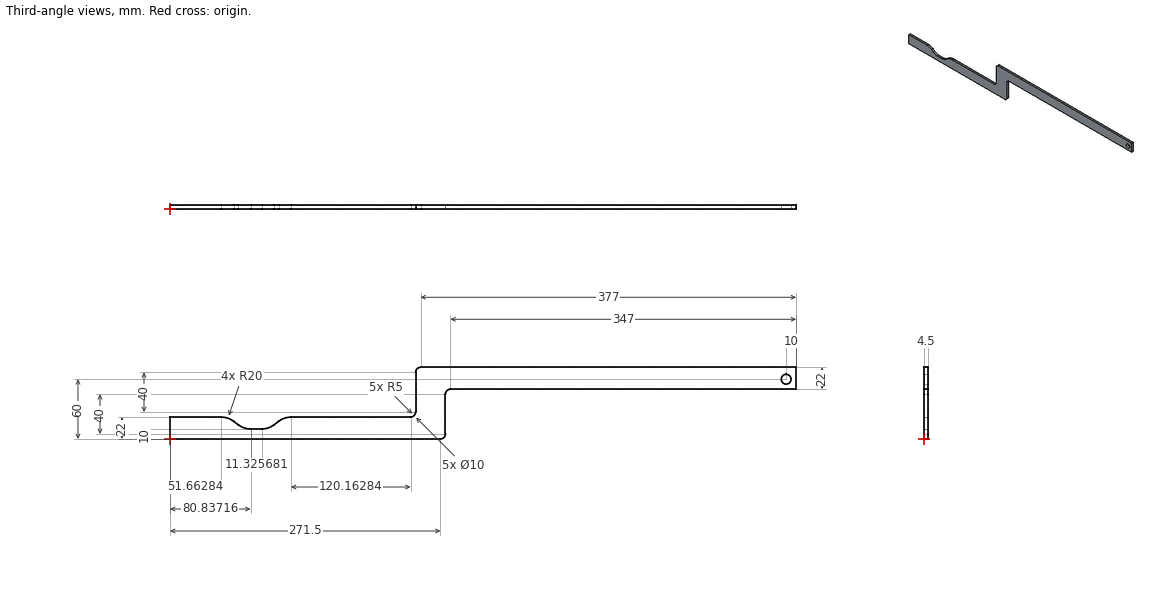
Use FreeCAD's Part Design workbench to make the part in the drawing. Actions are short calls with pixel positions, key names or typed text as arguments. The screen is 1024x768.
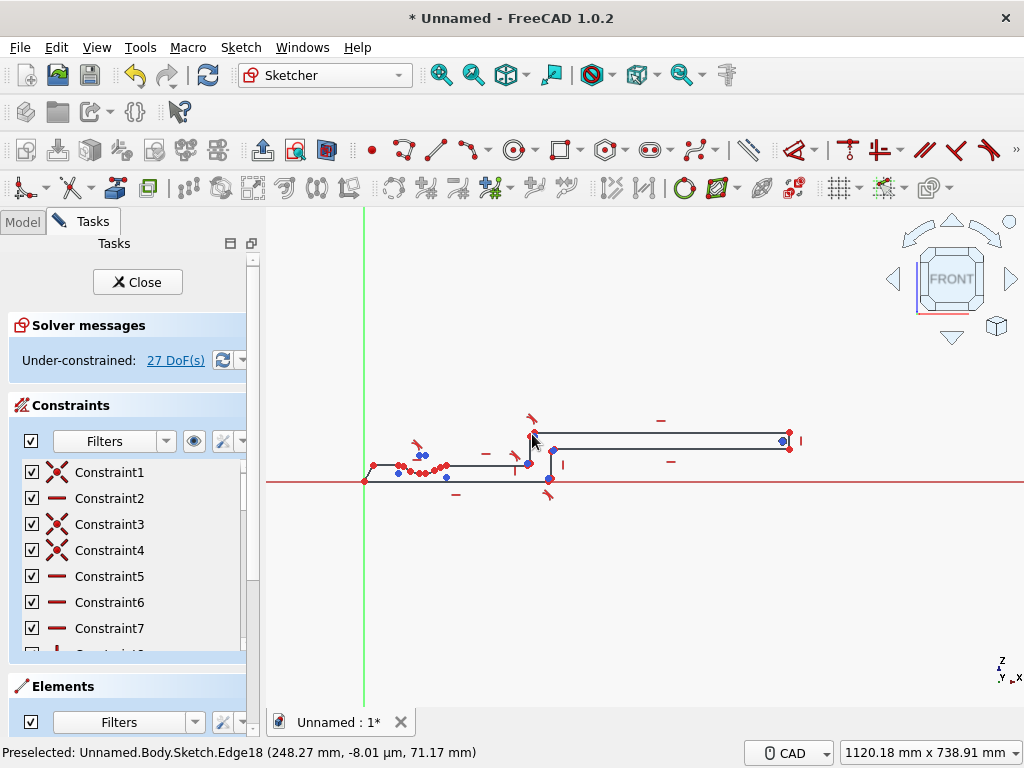
click(719, 449)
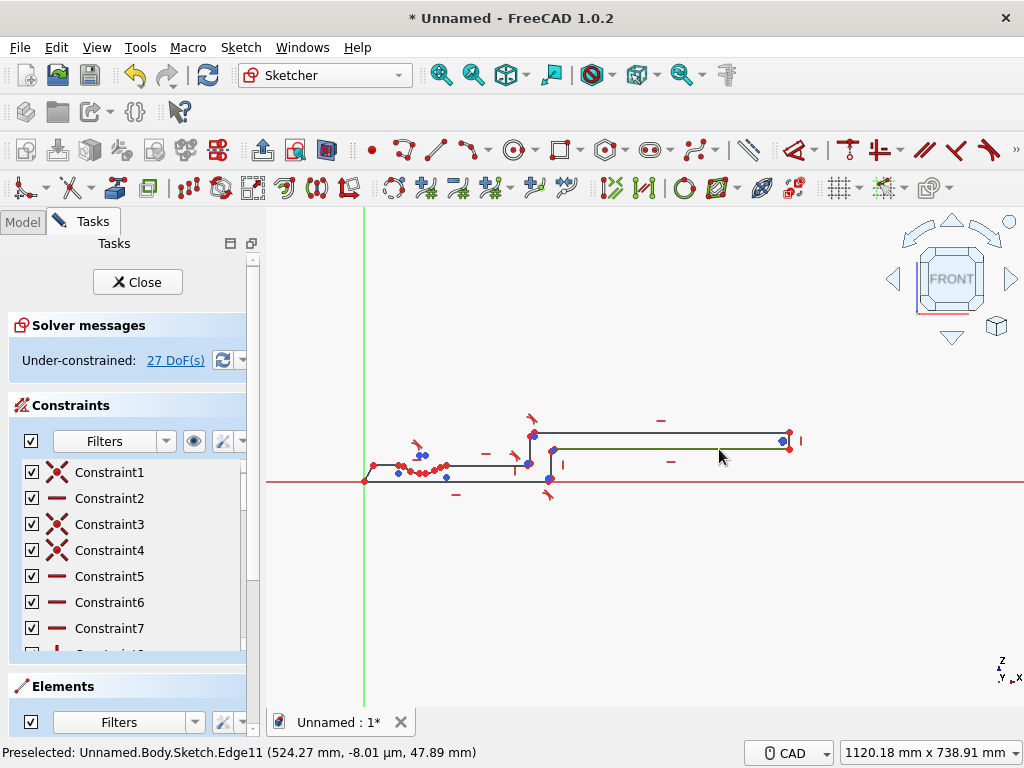
scroll(552, 449, up, 10)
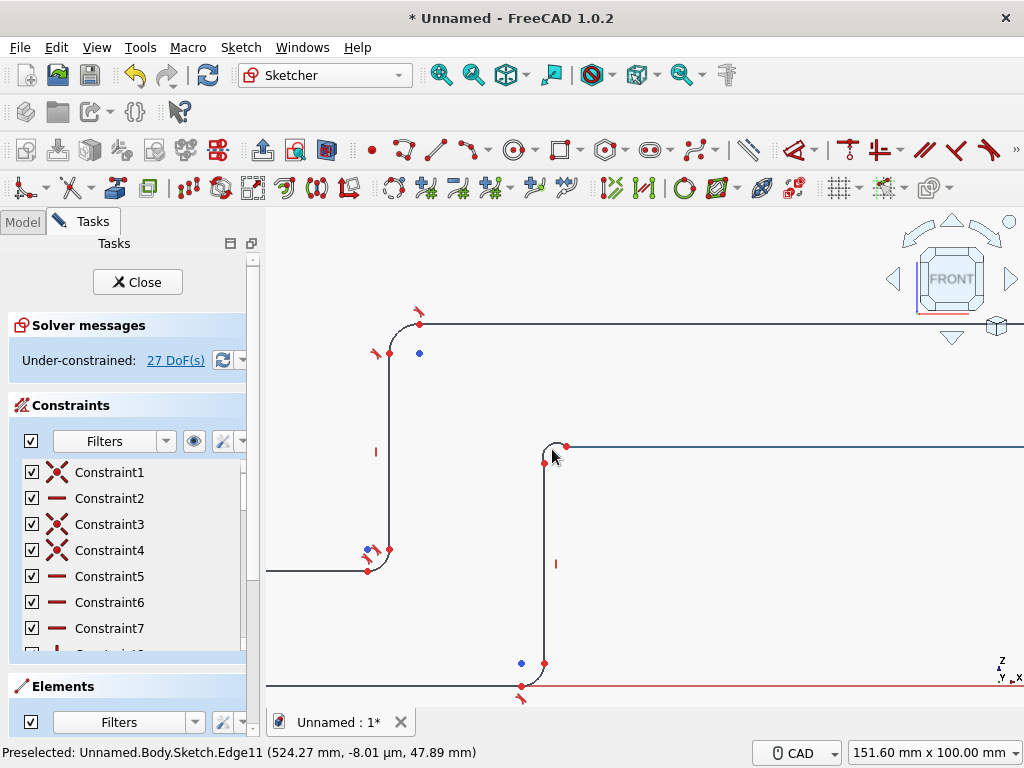
click(548, 446)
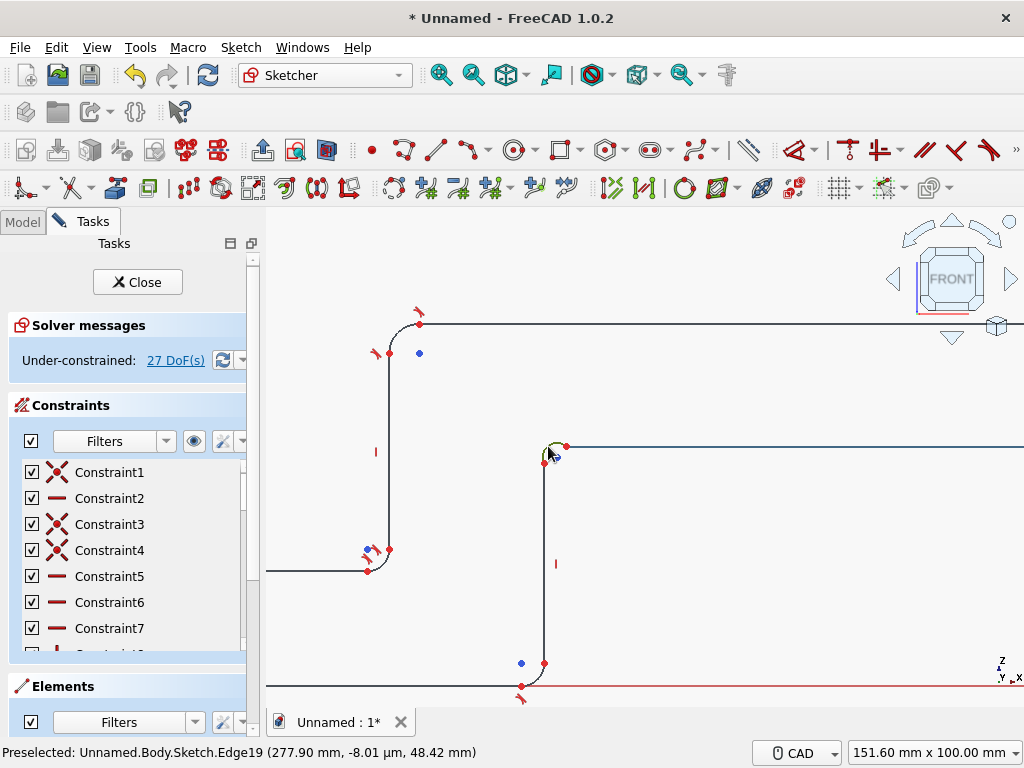
key(t)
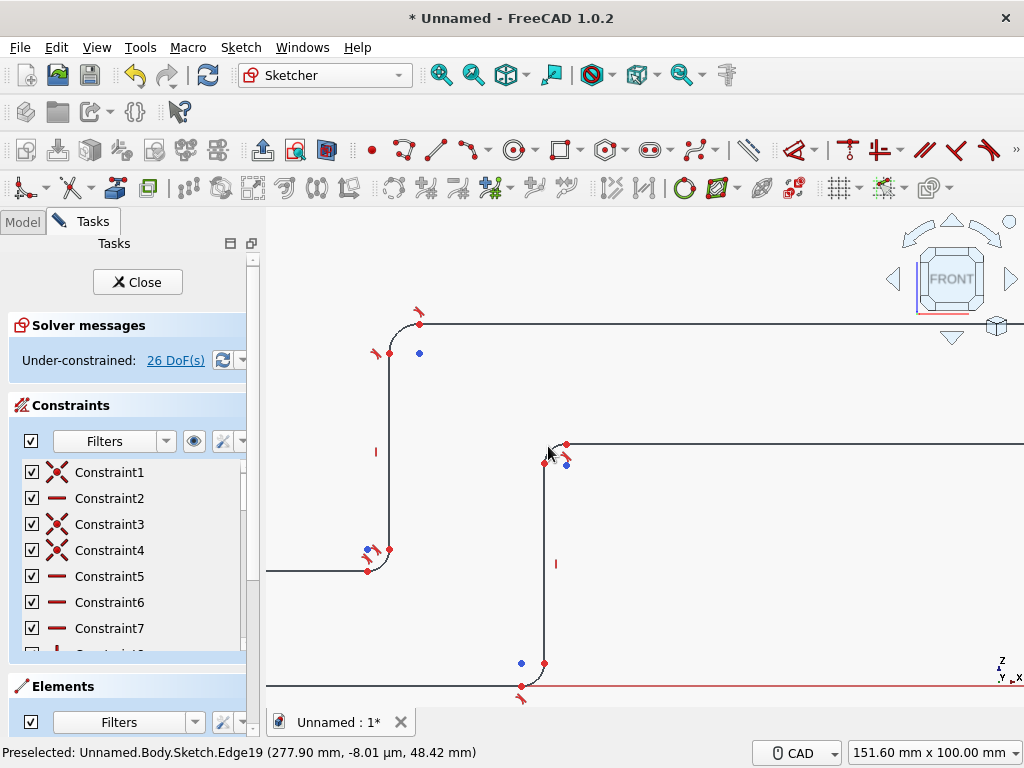
scroll(552, 449, down, 10)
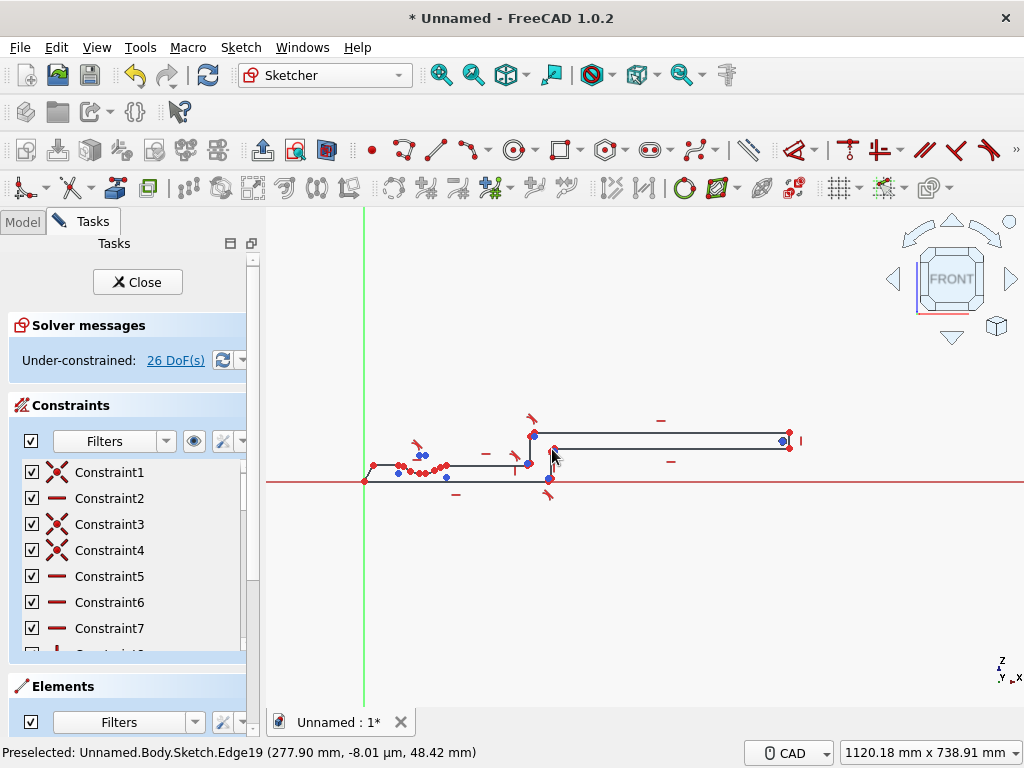
scroll(551, 460, up, 3)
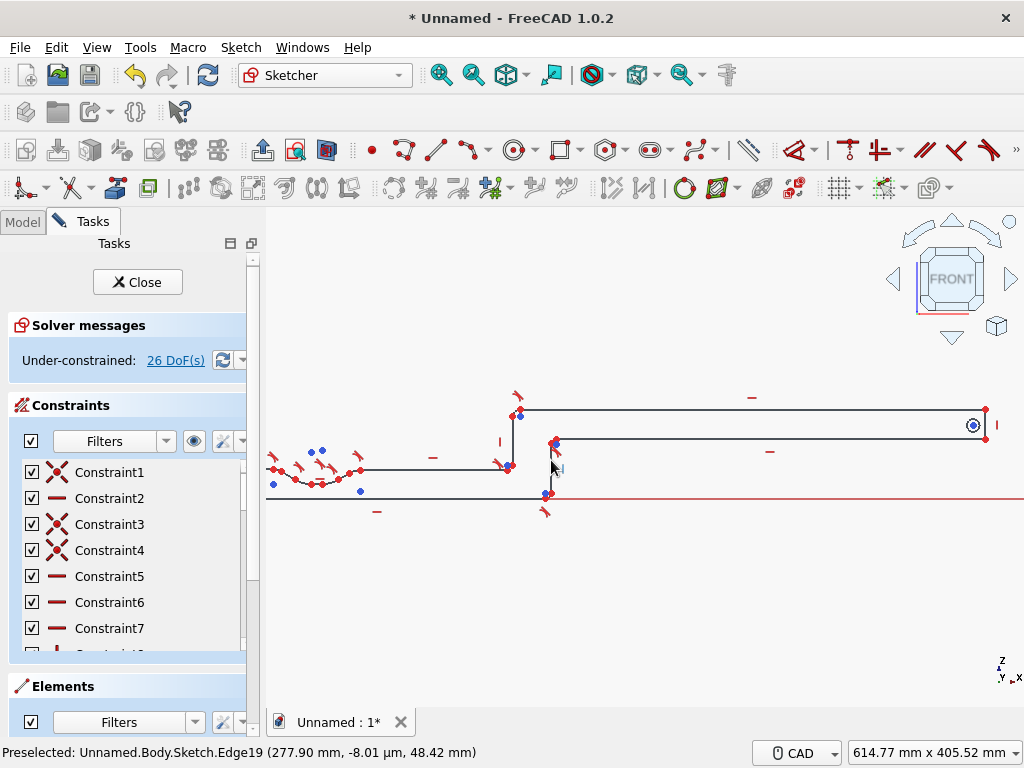
click(551, 459)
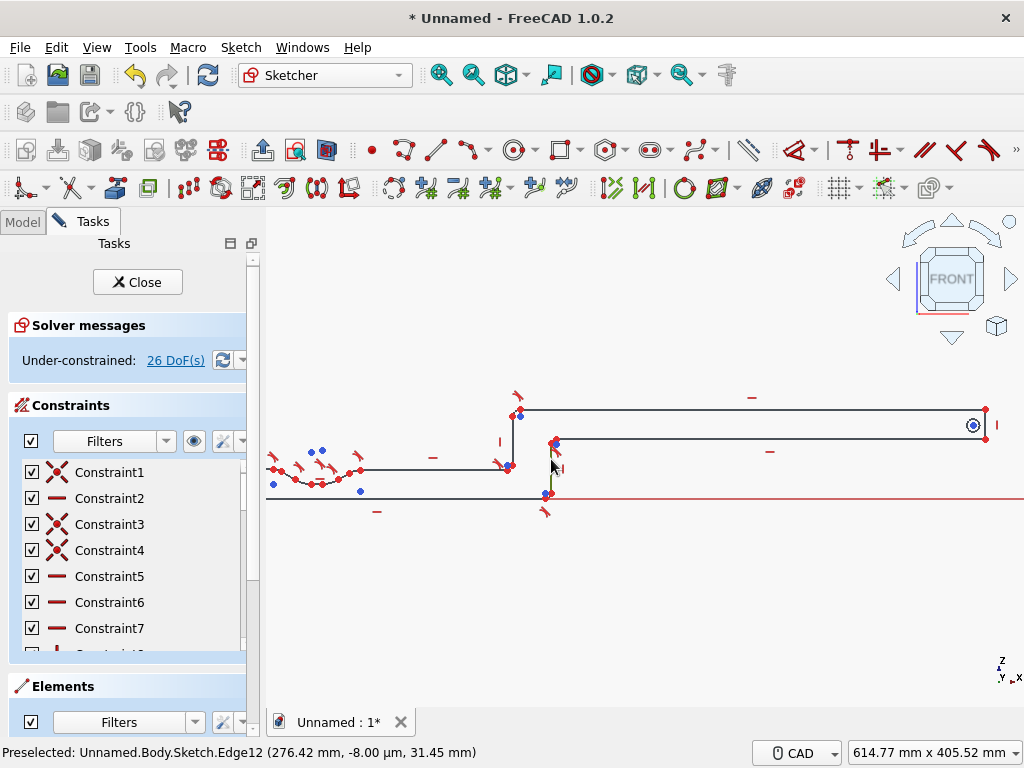
scroll(553, 440, up, 7)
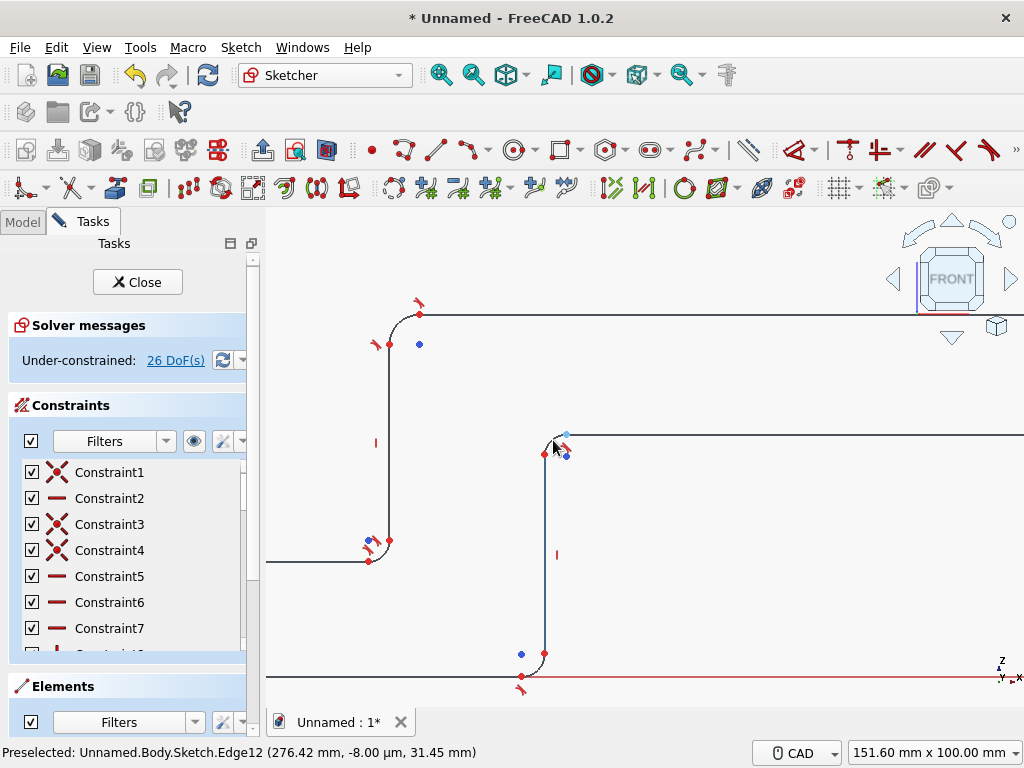
click(552, 441)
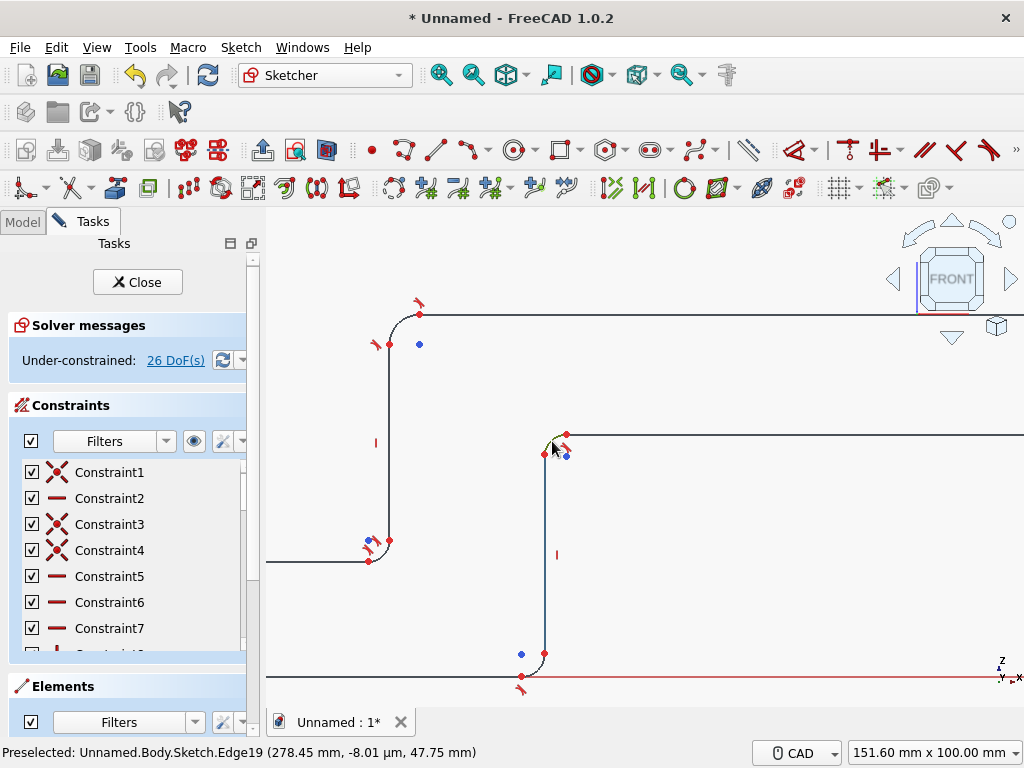
click(990, 150)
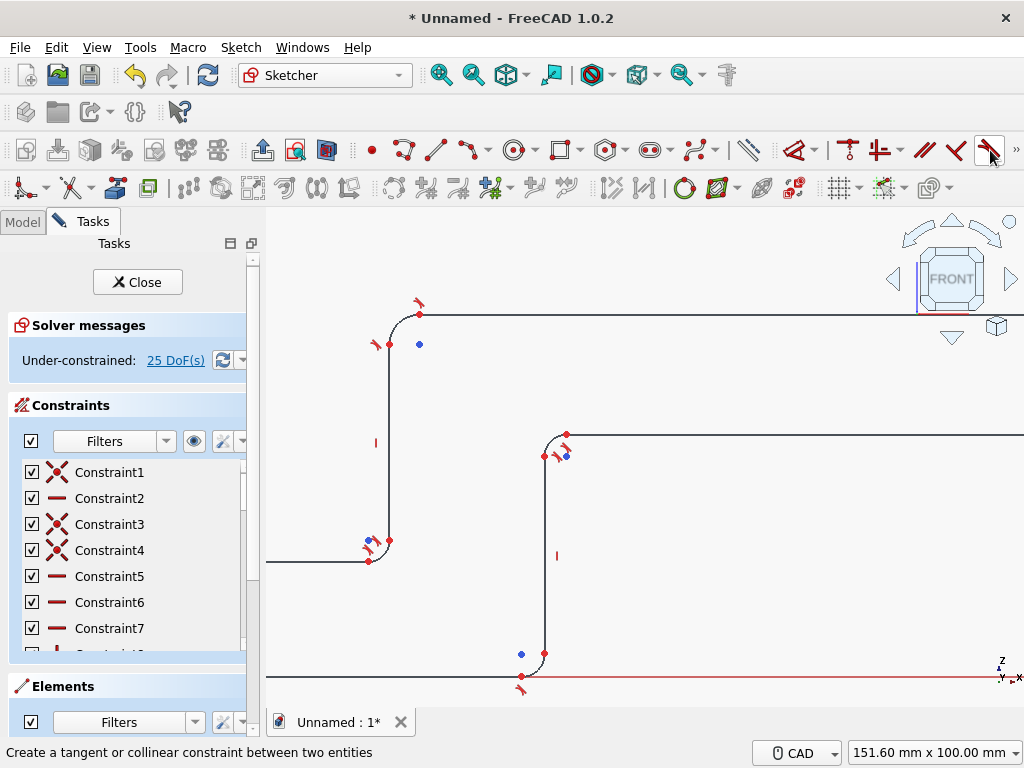
scroll(552, 451, down, 10)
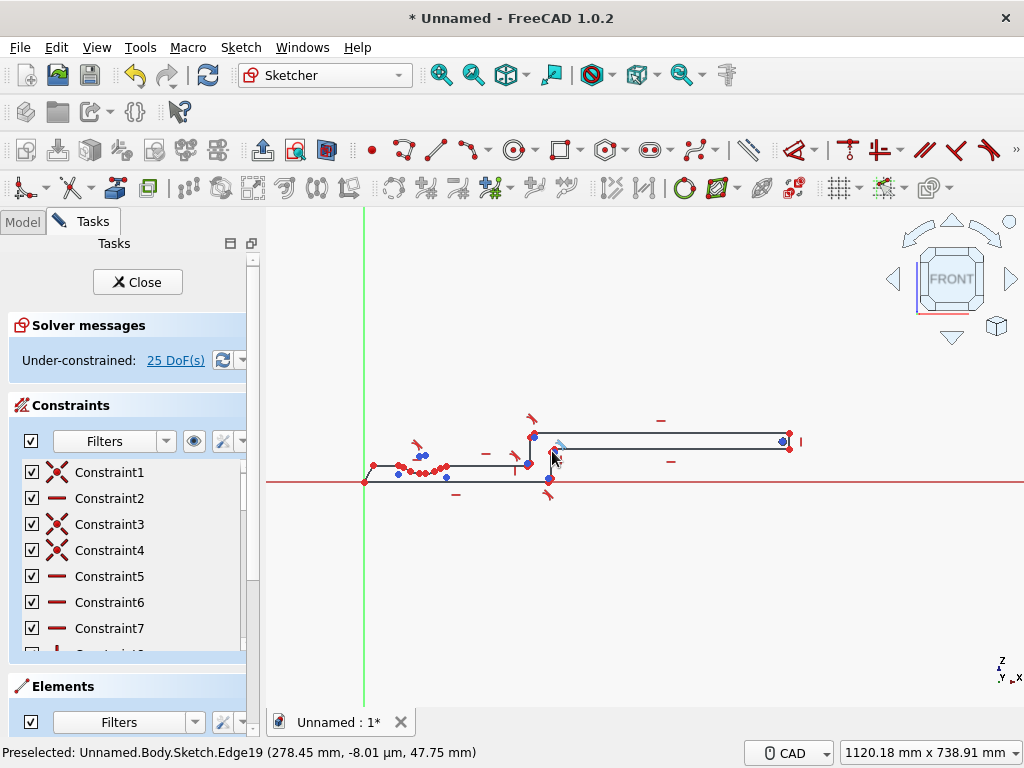
scroll(551, 460, up, 3)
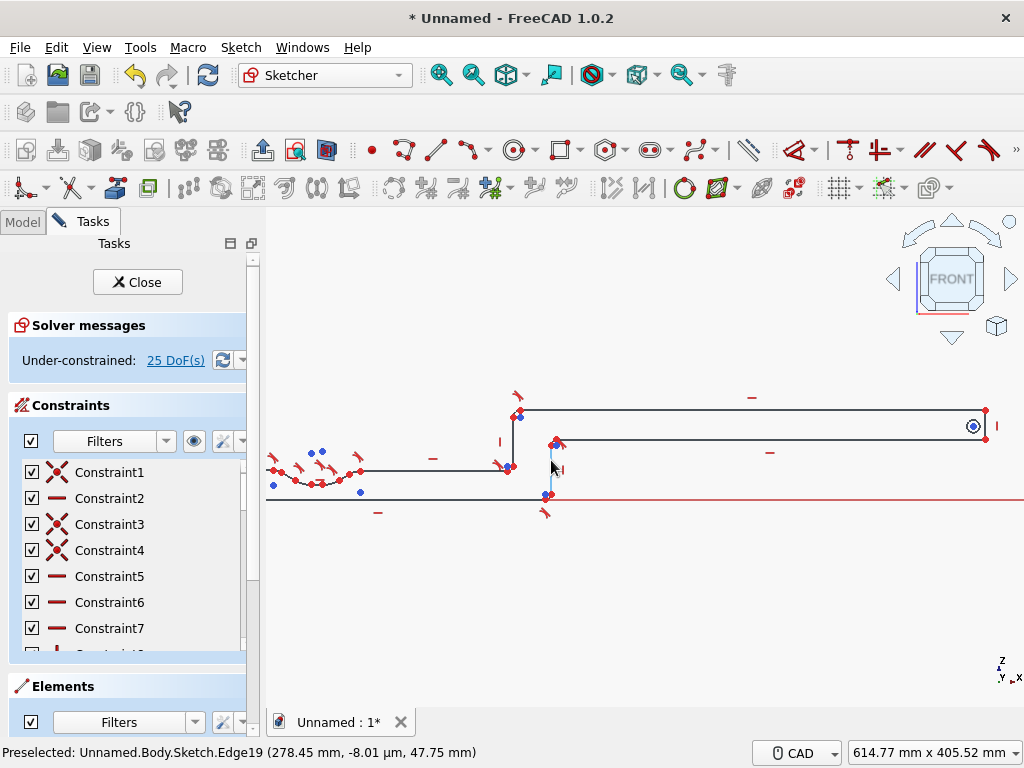
click(551, 460)